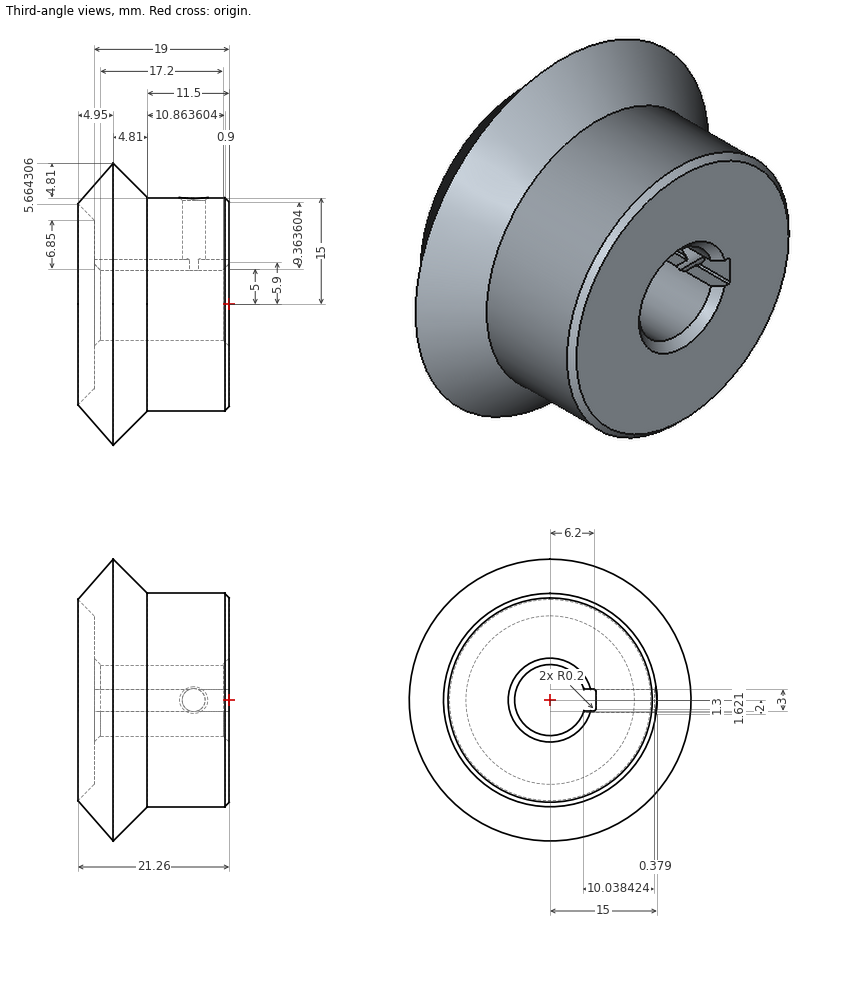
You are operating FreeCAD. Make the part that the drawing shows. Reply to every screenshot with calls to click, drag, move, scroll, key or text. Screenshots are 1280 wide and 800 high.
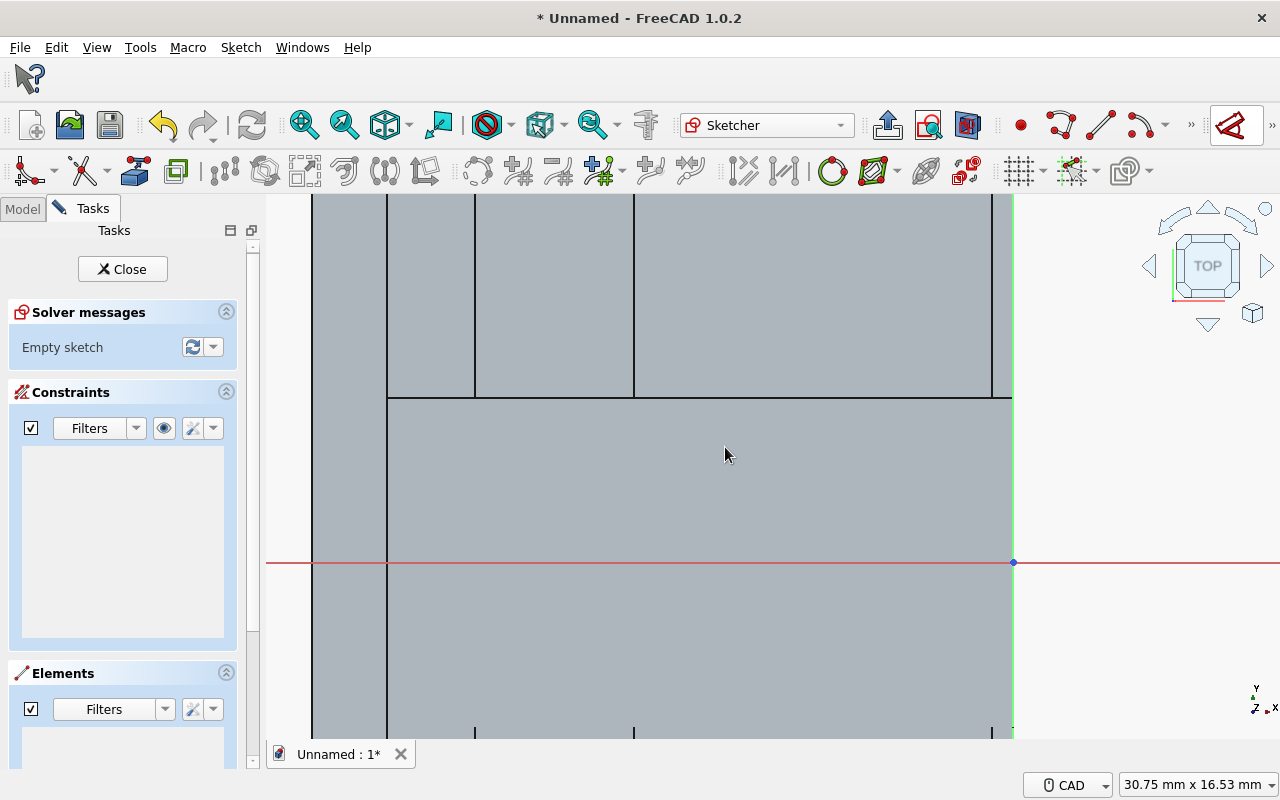
click(1062, 126)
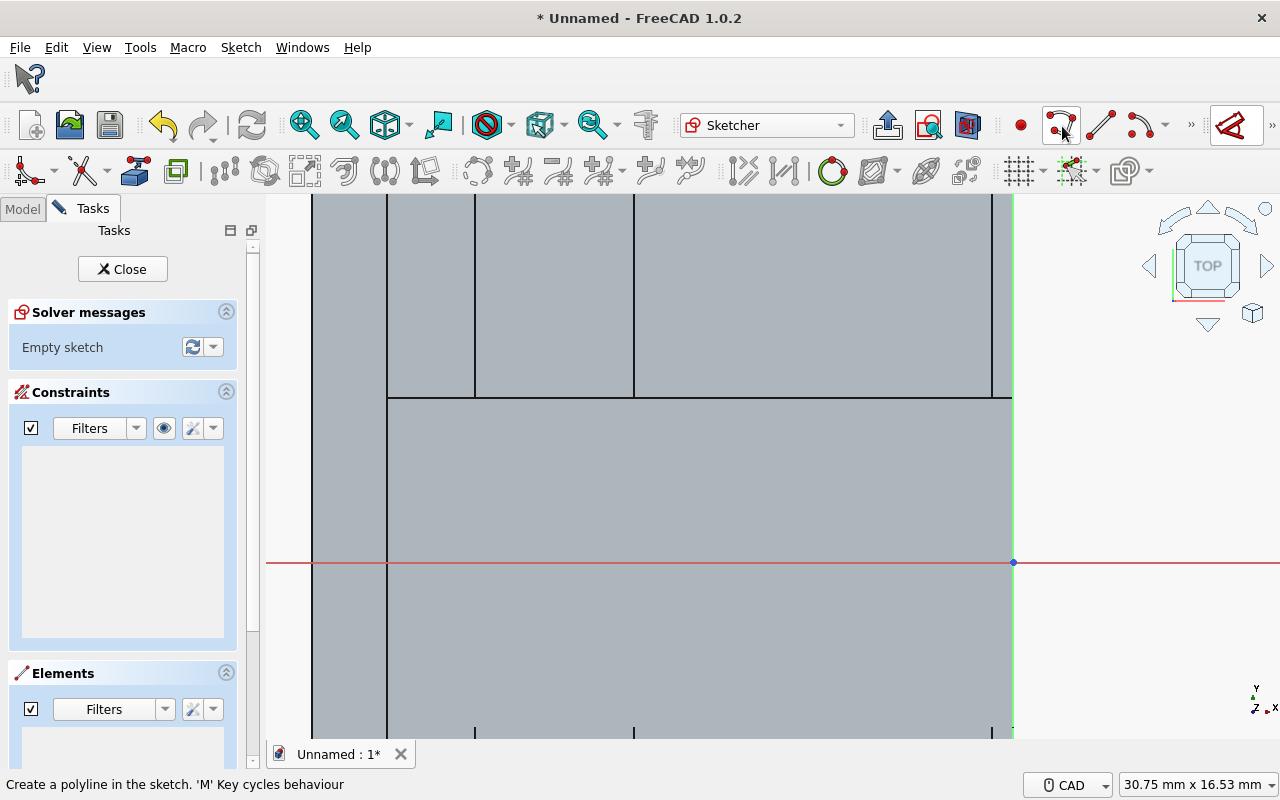
click(1013, 563)
click(1004, 368)
click(983, 398)
click(416, 398)
click(387, 368)
click(387, 554)
click(1013, 563)
key(Escape)
key(Escape)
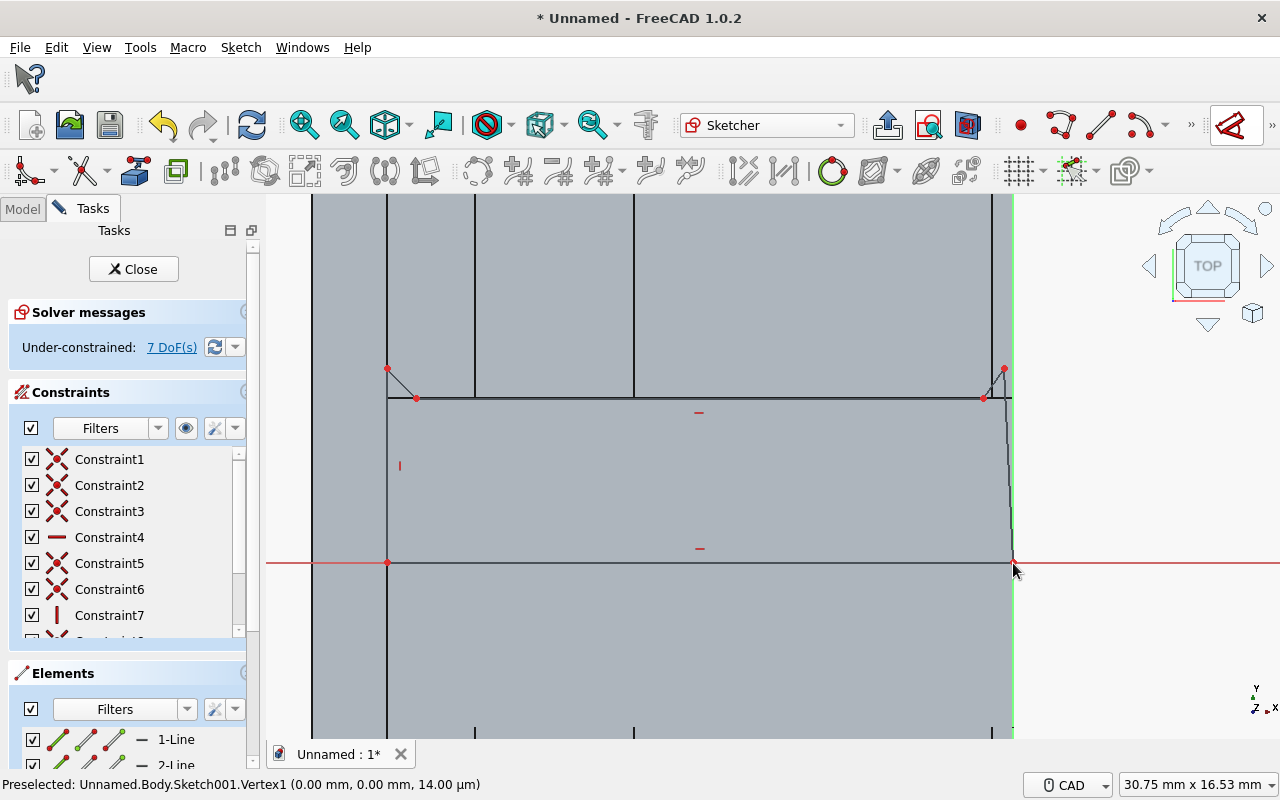
click(1010, 505)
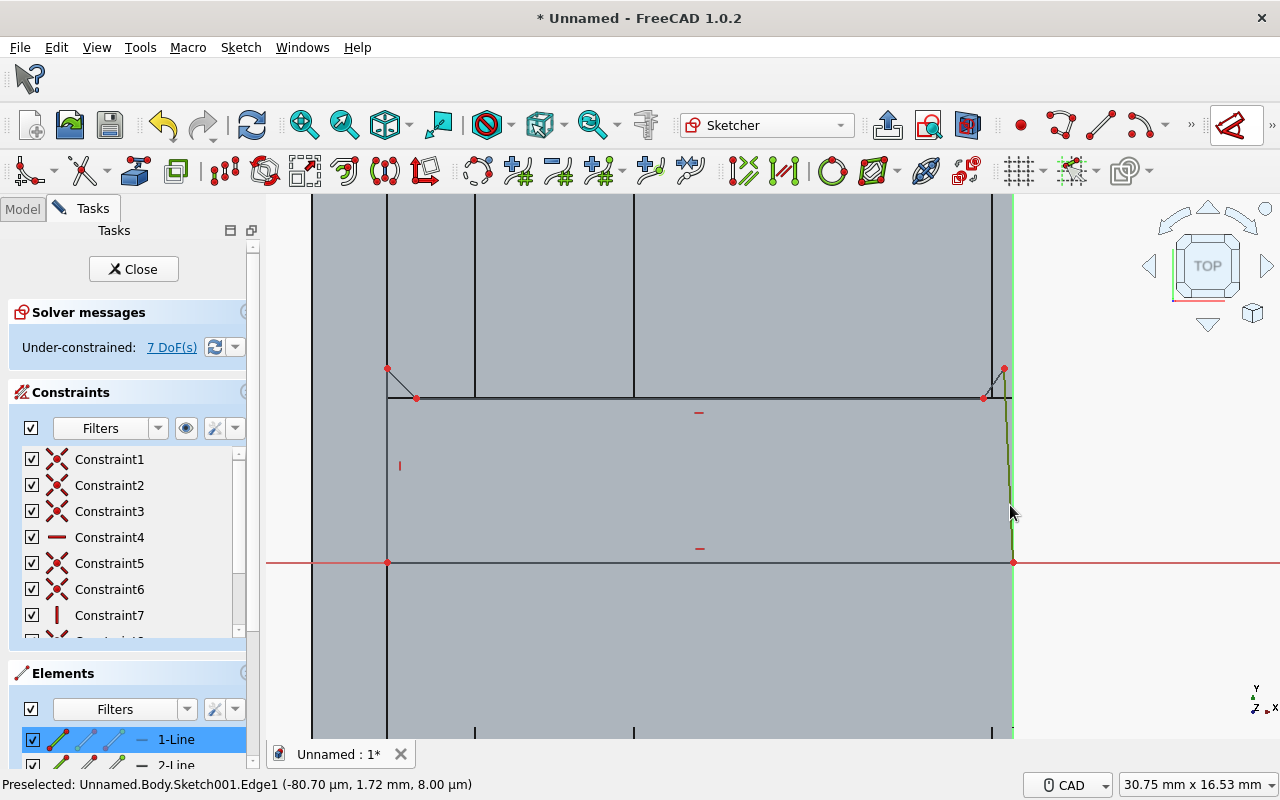
key(v)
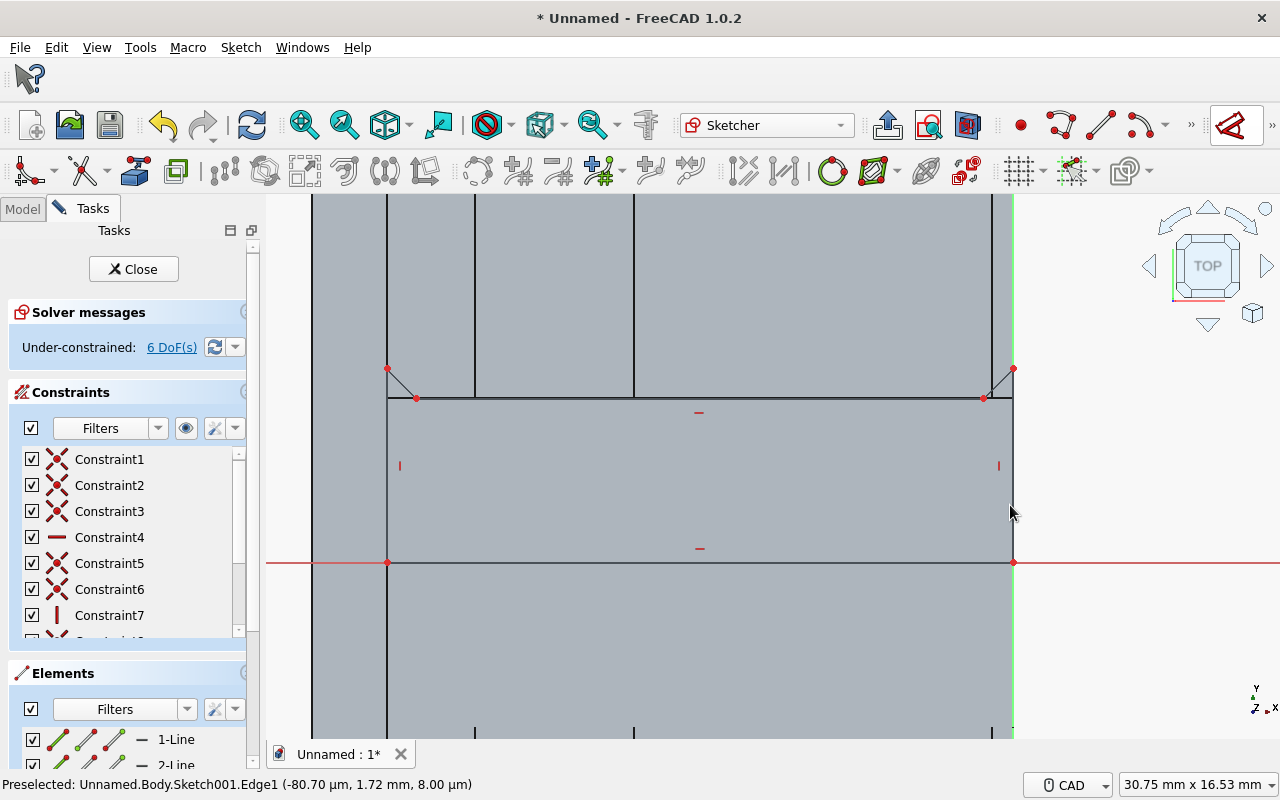
click(575, 563)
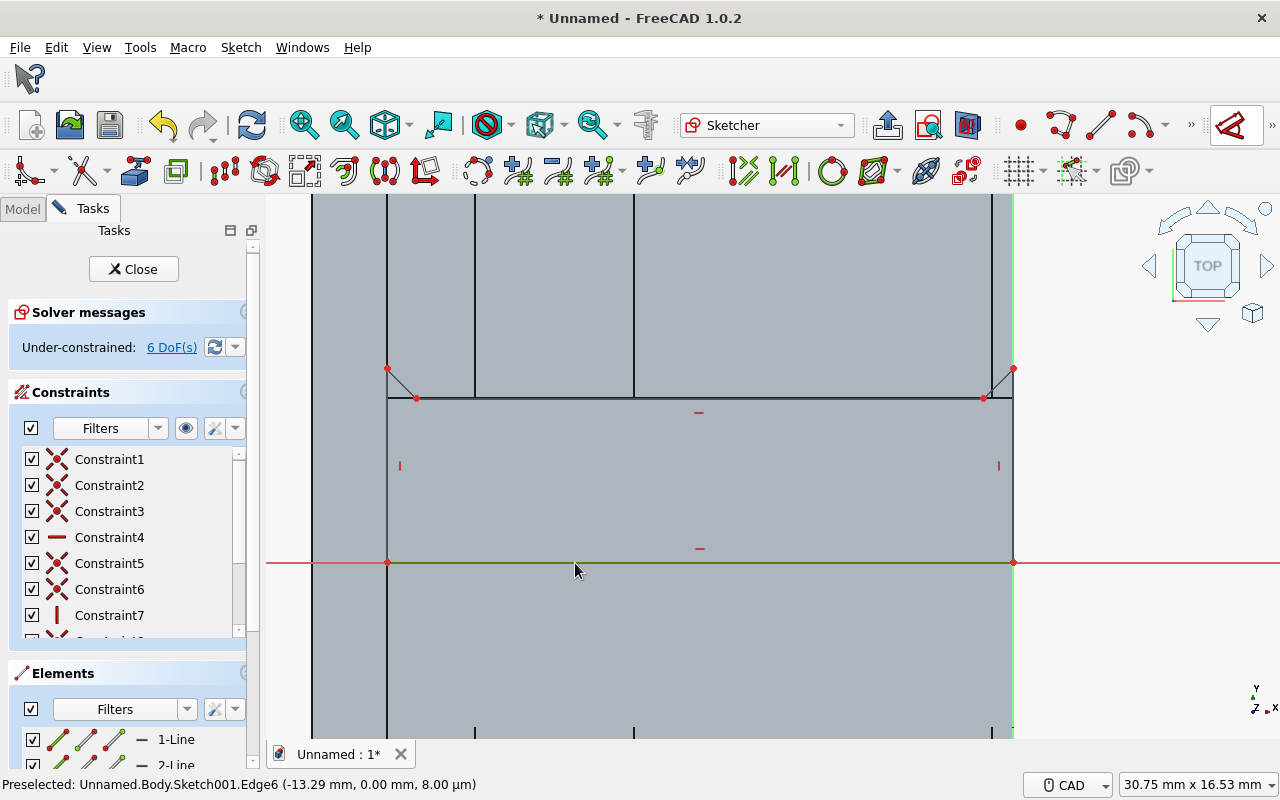
key(l)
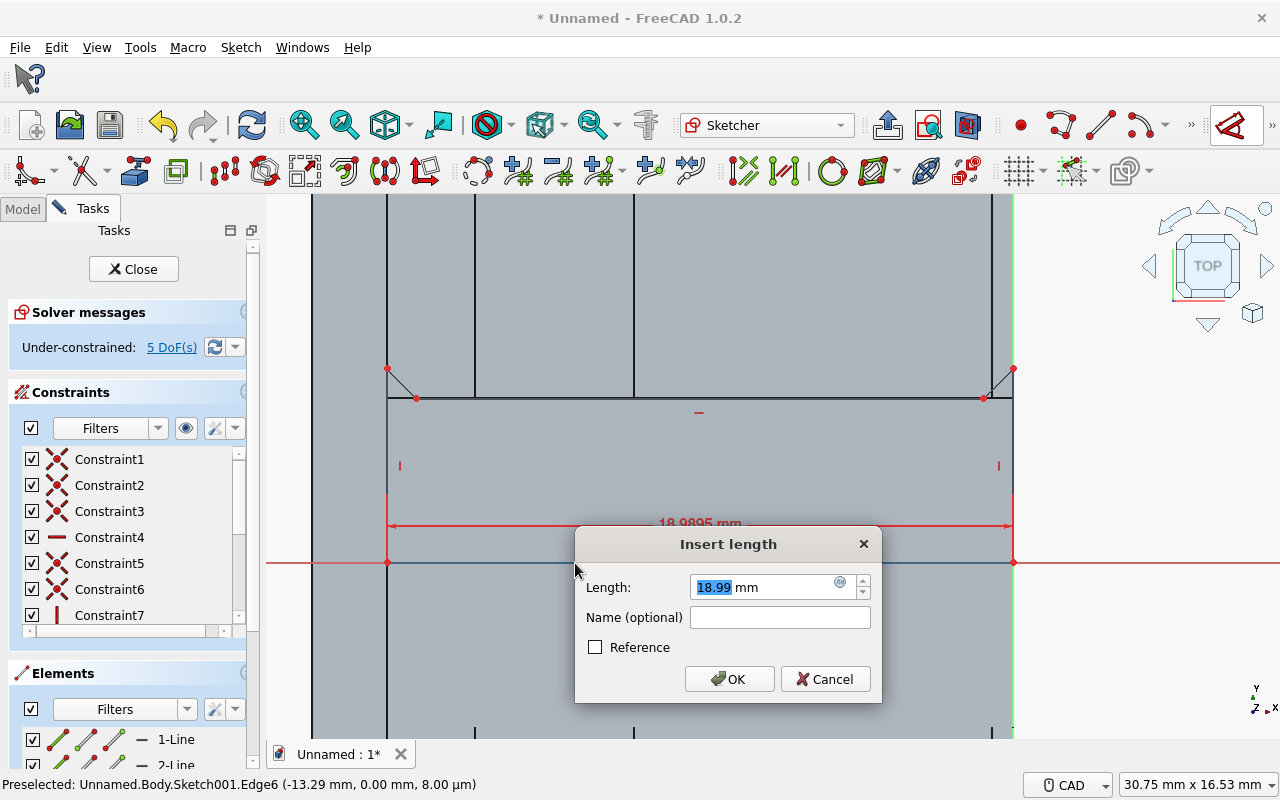
text(19)
key(Return)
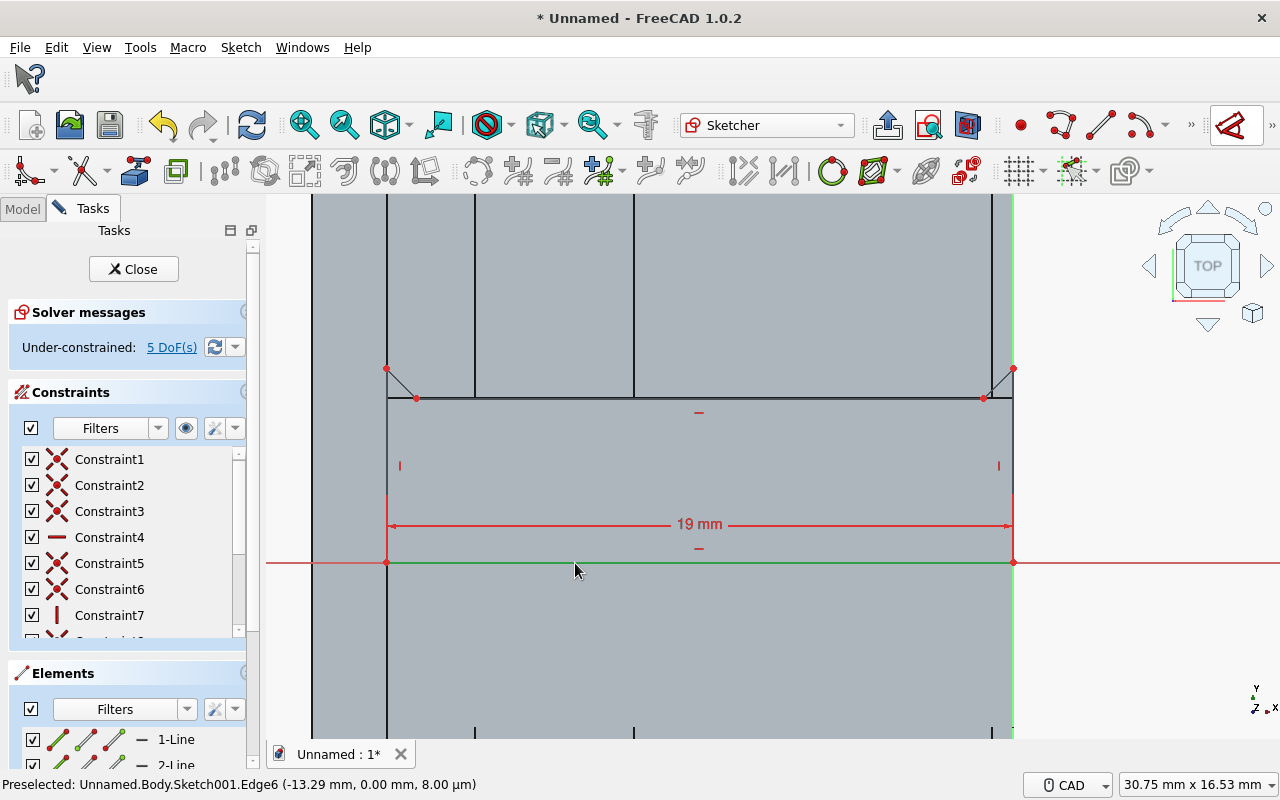
click(983, 399)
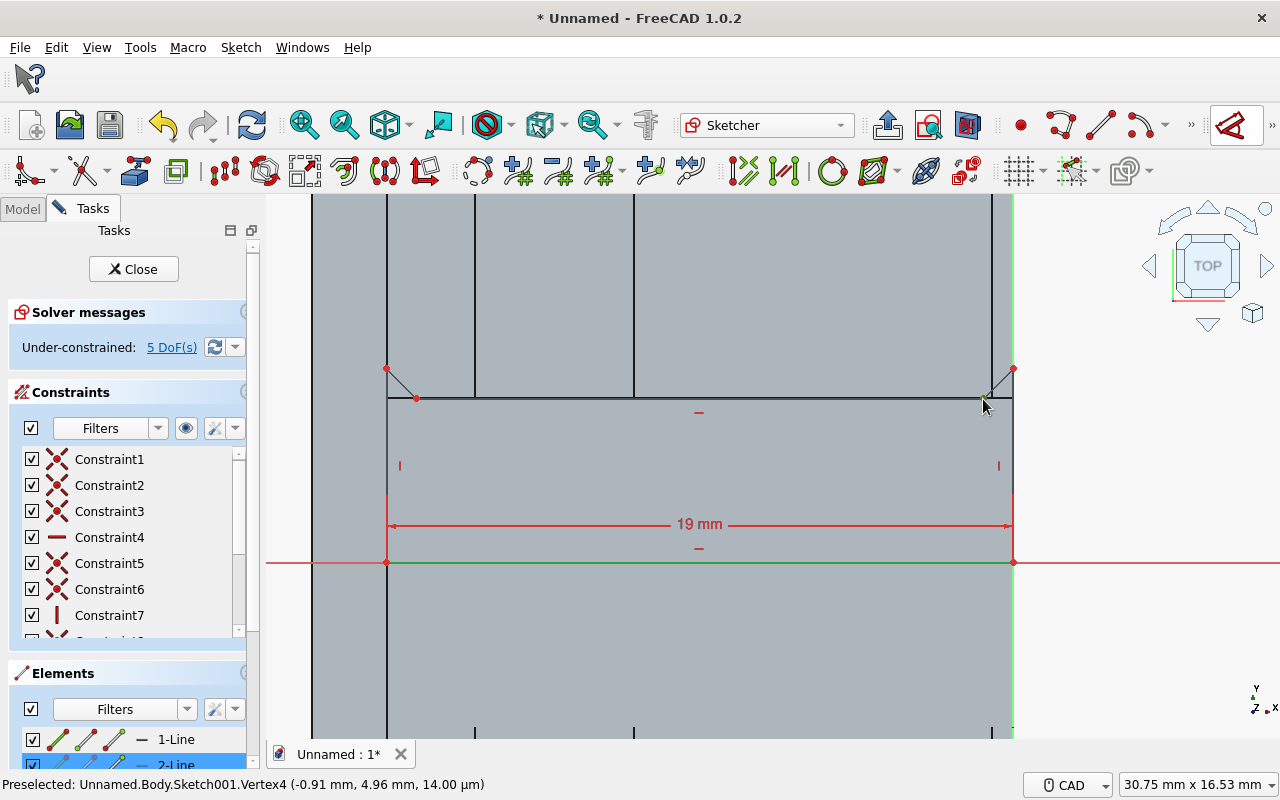
click(1258, 126)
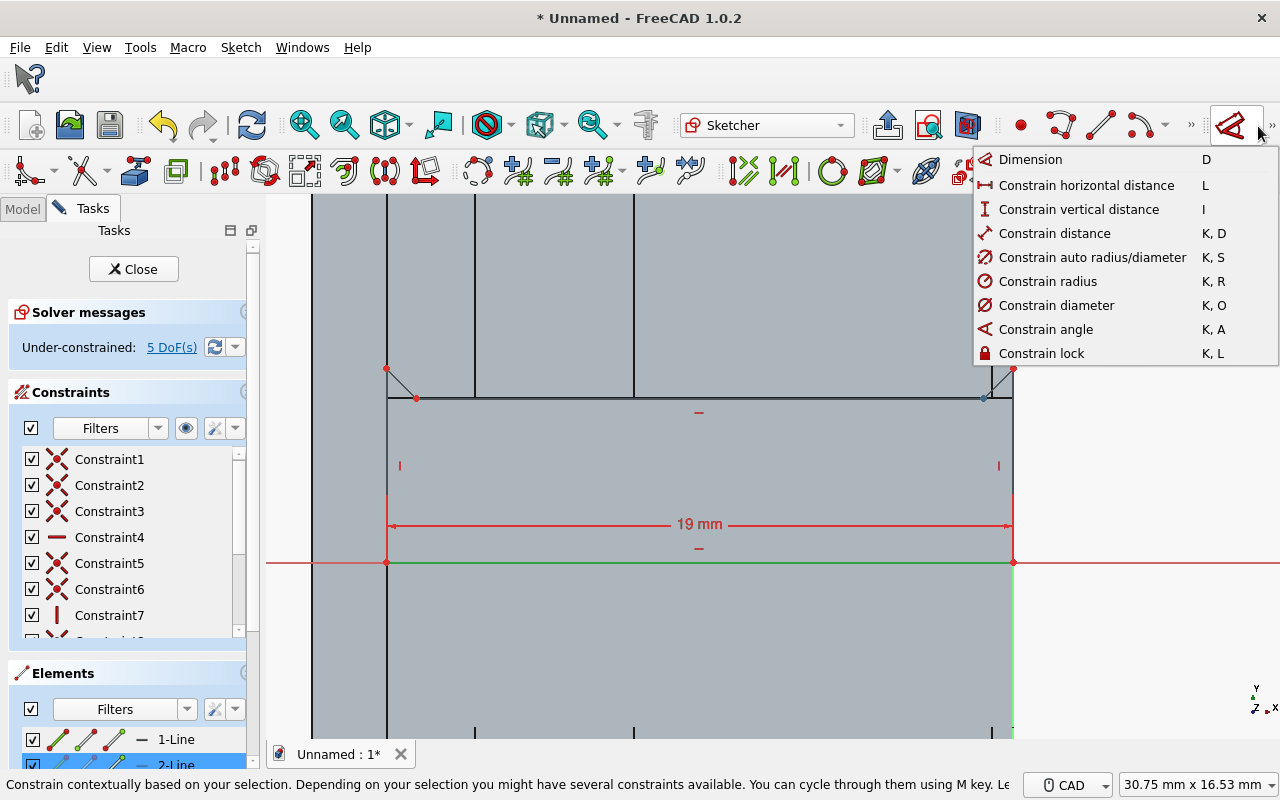
click(1126, 209)